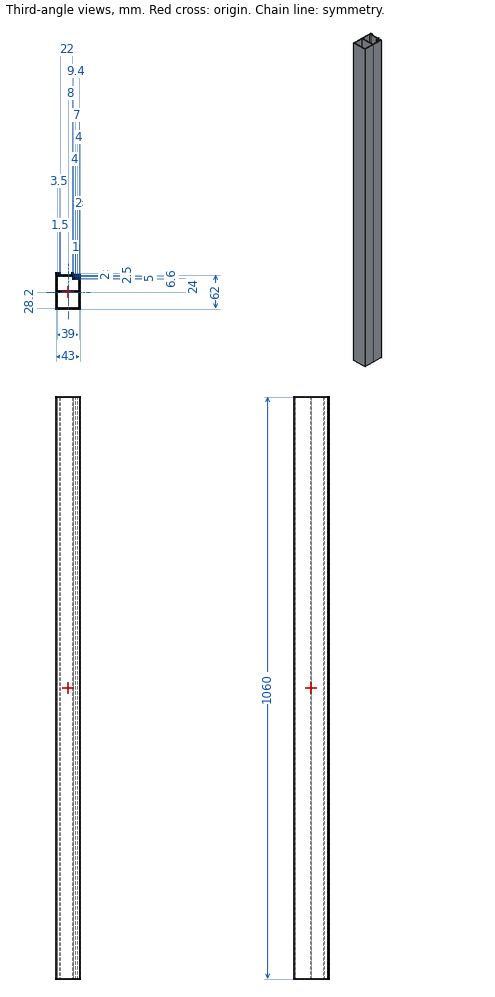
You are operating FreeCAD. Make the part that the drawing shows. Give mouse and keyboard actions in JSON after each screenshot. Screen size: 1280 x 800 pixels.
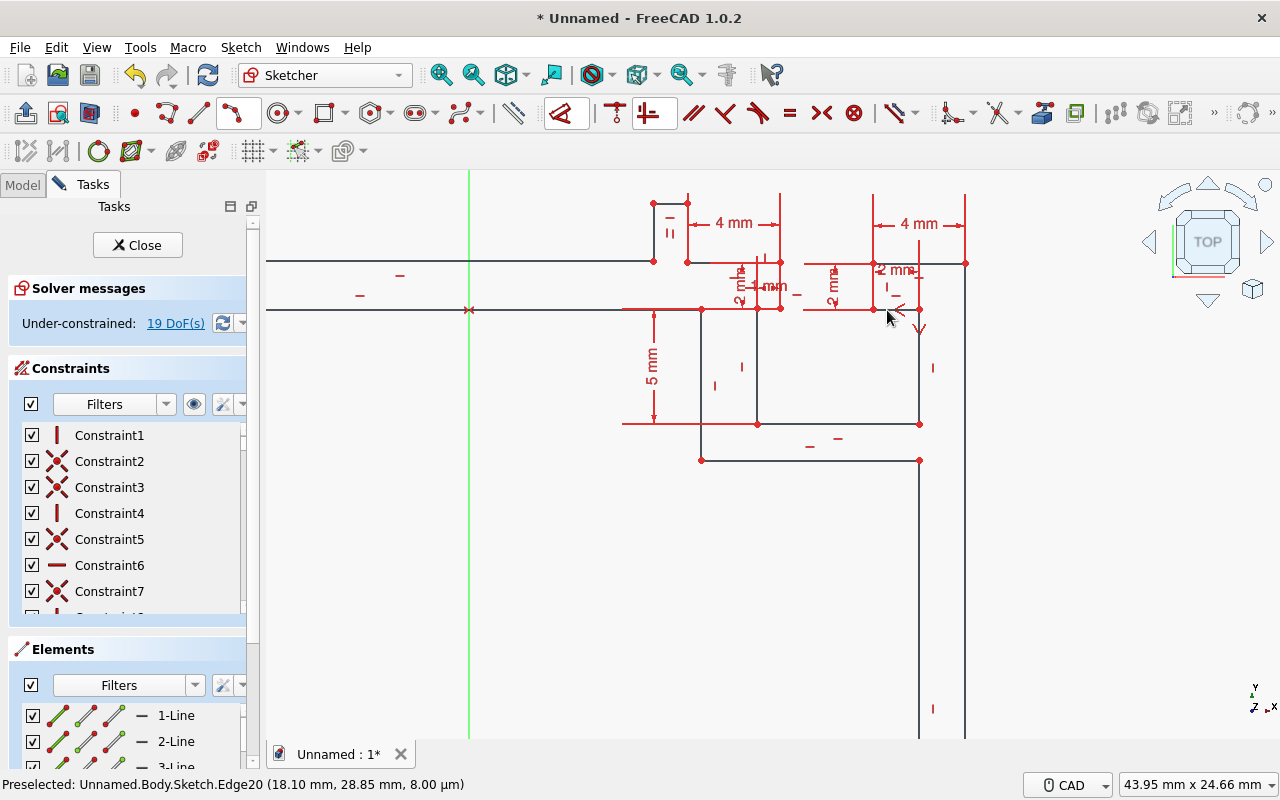
{"action": "left_click", "coordinate": [919, 344]}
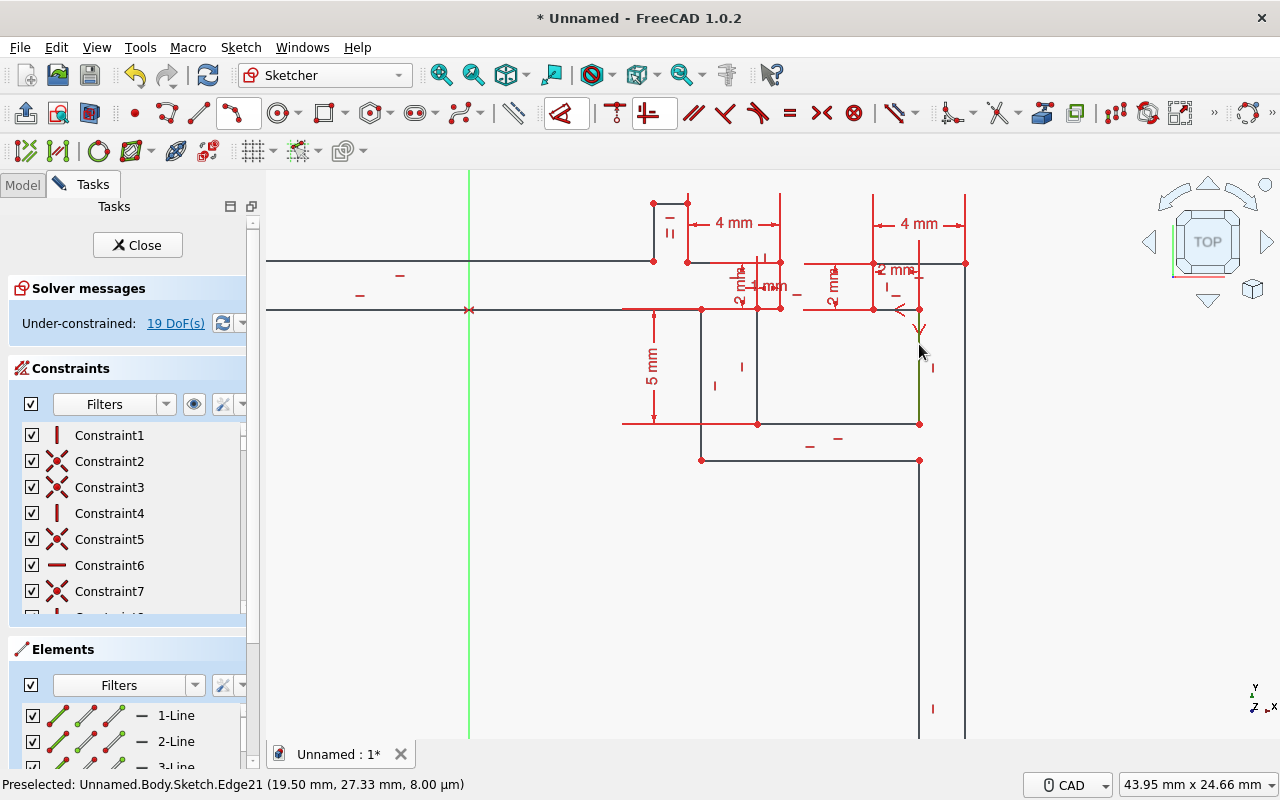
{"action": "key", "text": "i"}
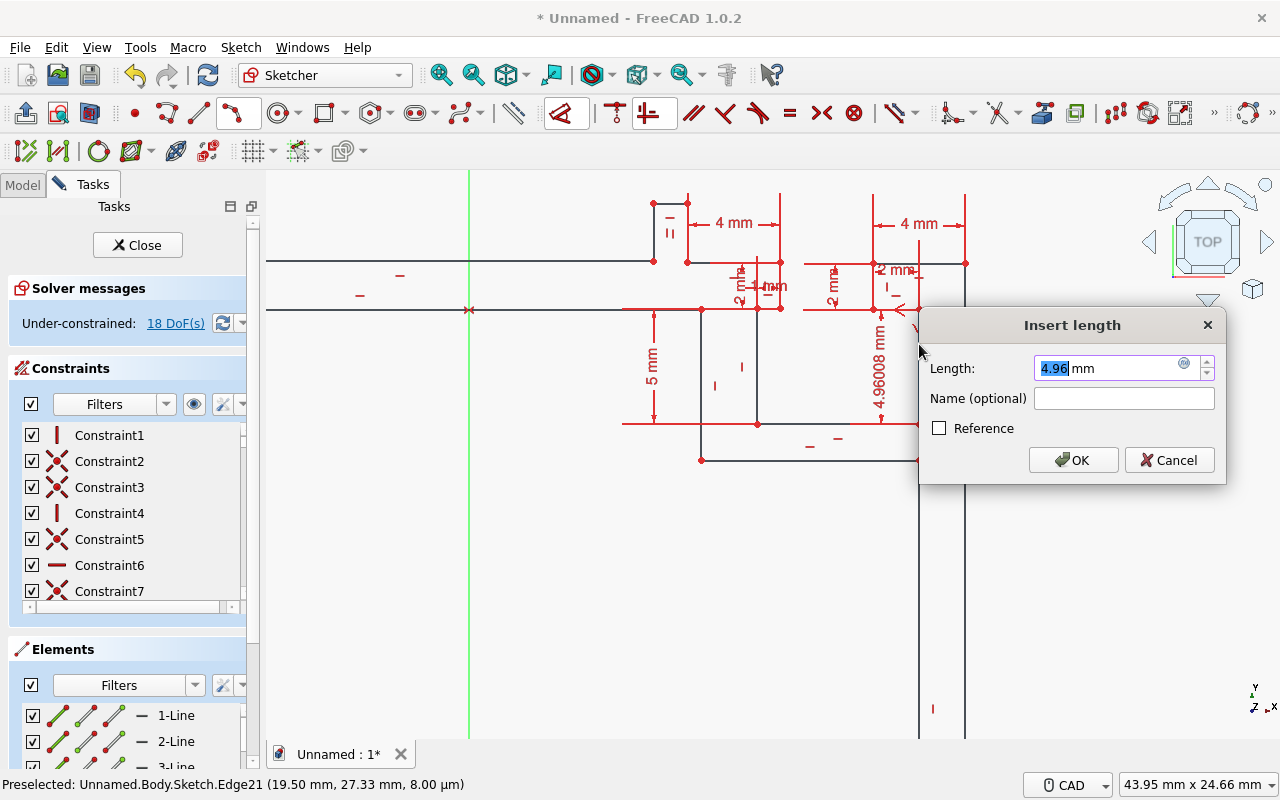
{"action": "type", "text": "5"}
{"action": "key", "text": "Return"}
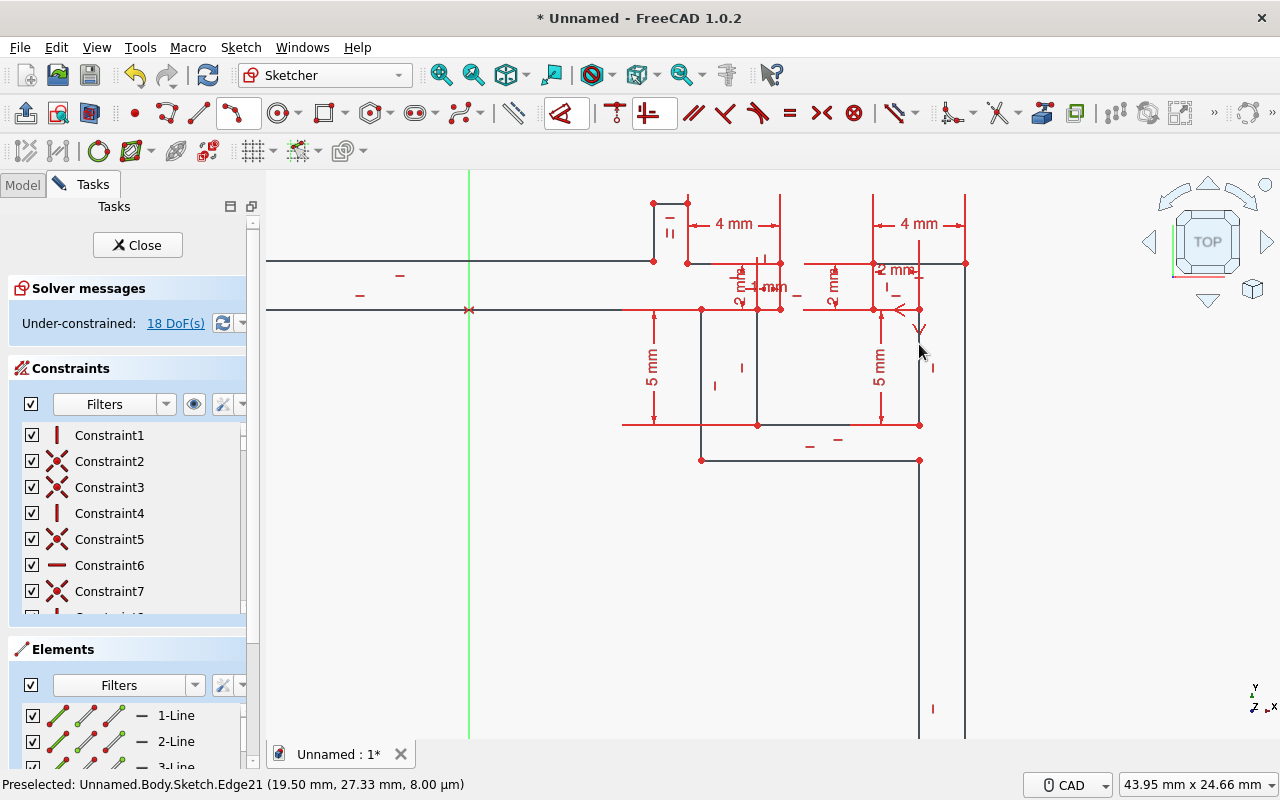
{"action": "left_click", "coordinate": [871, 425]}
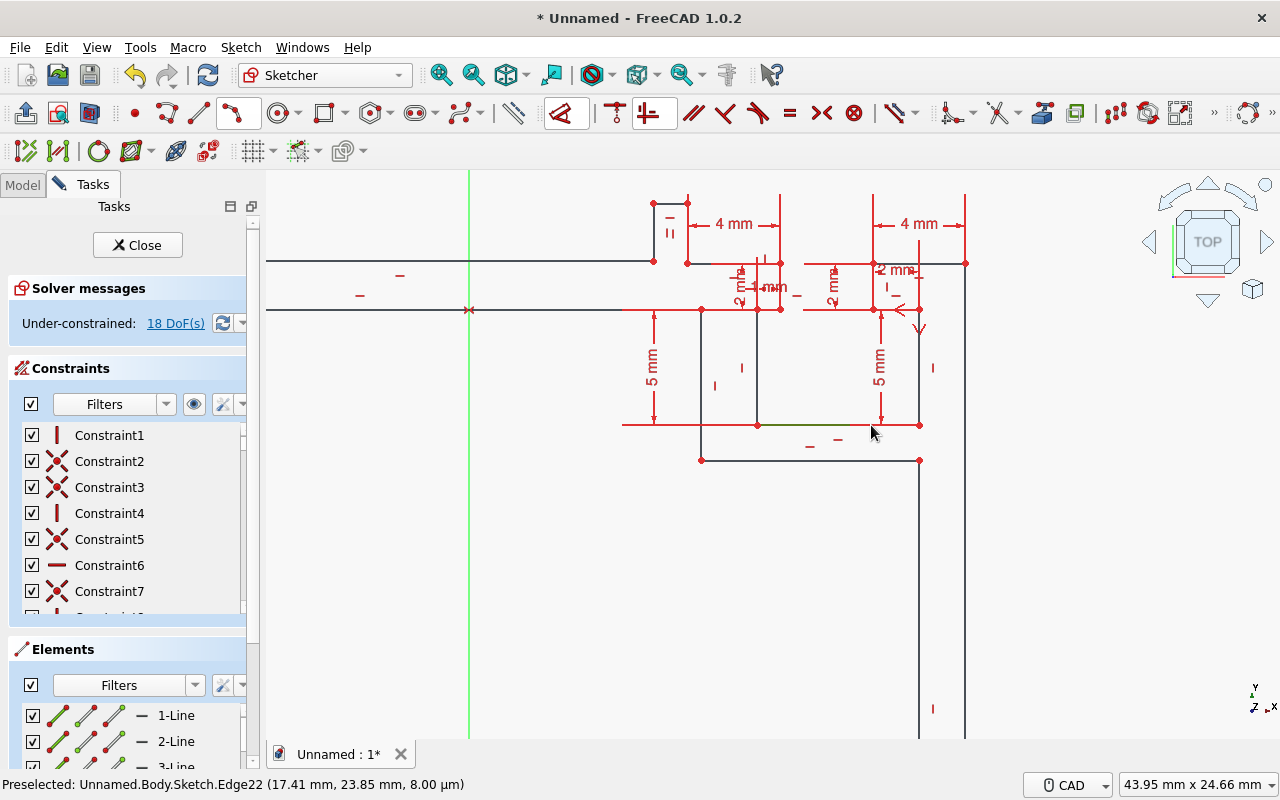
{"action": "left_click", "coordinate": [584, 114]}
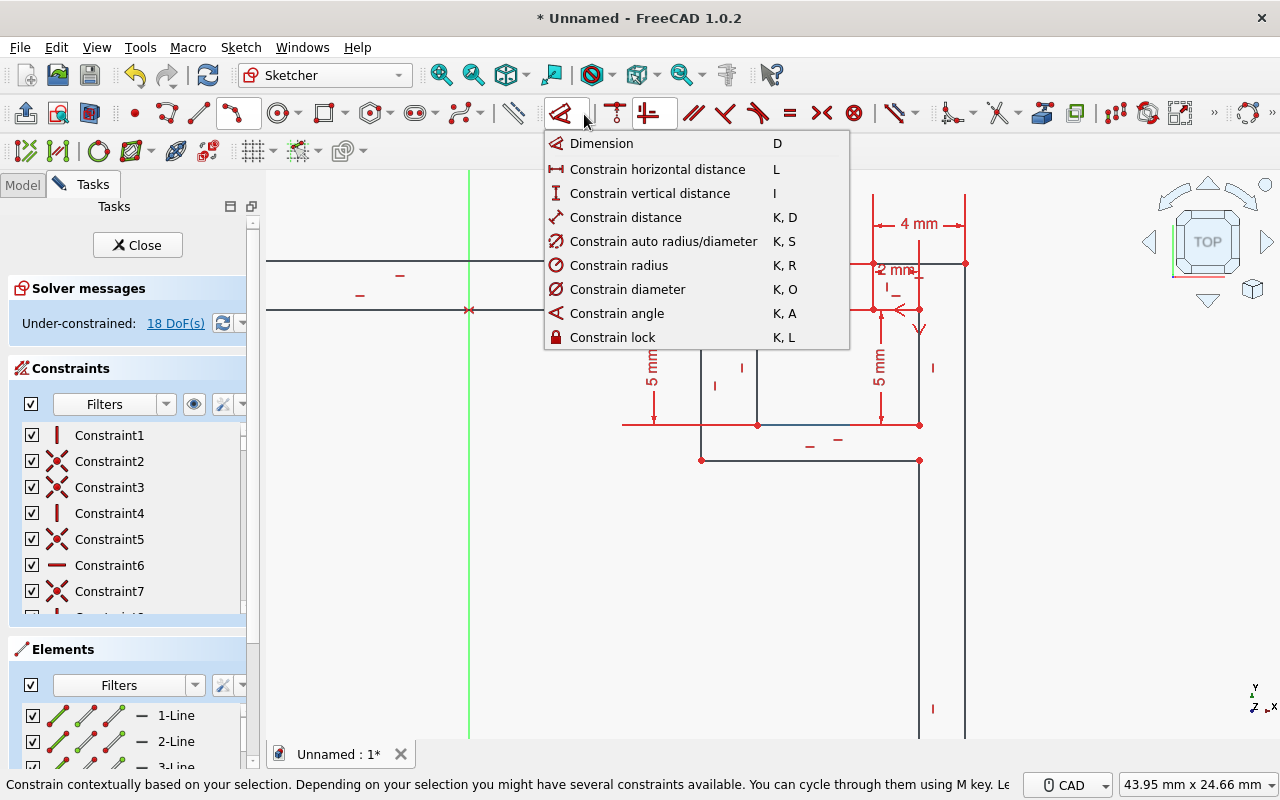
{"action": "left_click", "coordinate": [697, 169]}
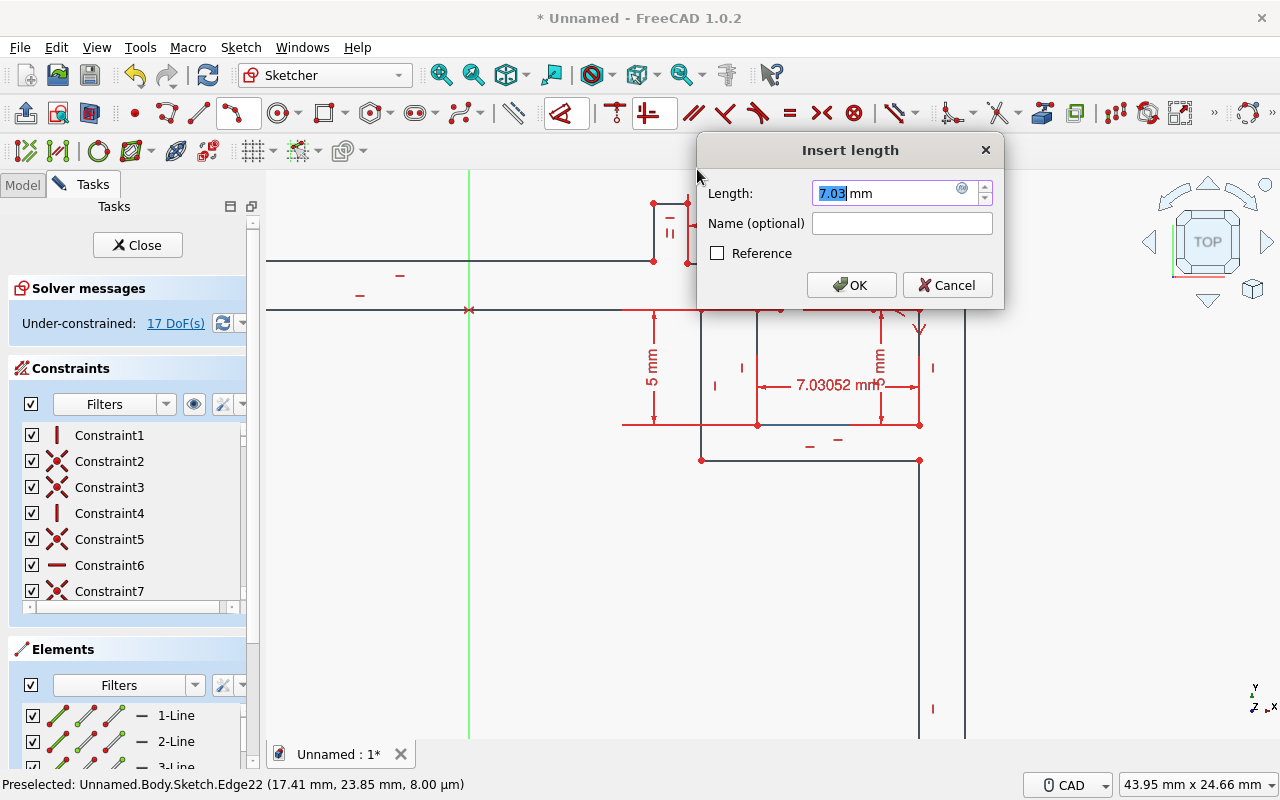
{"action": "type", "text": "7"}
{"action": "key", "text": "Return"}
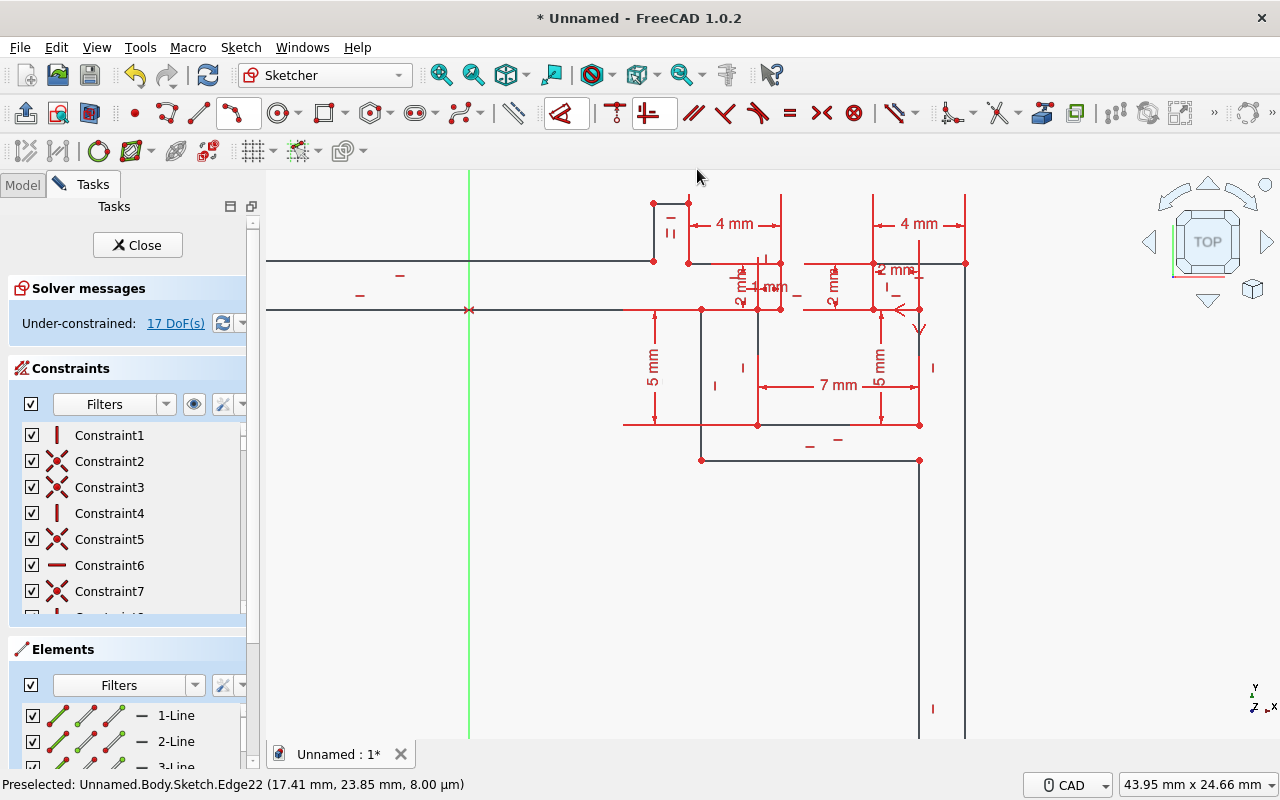
{"action": "left_click", "coordinate": [502, 261]}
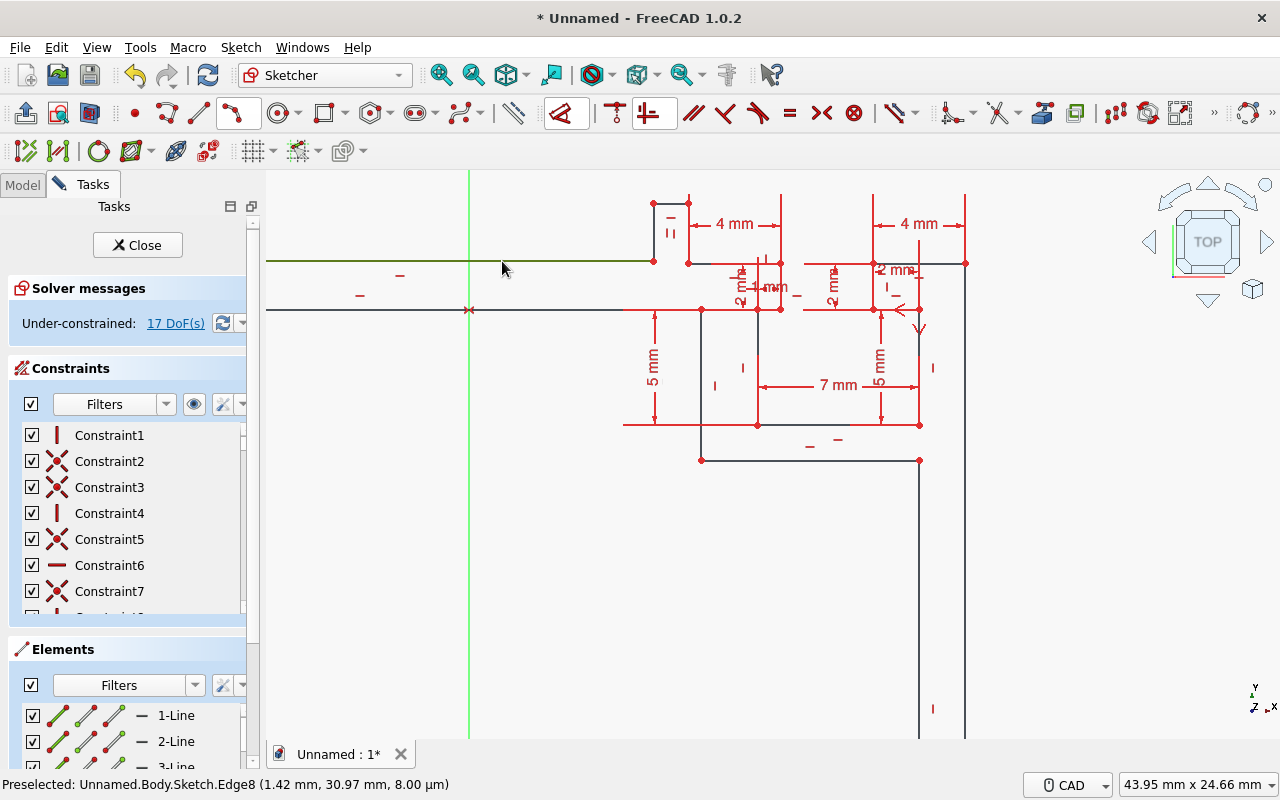
{"action": "key", "text": "l"}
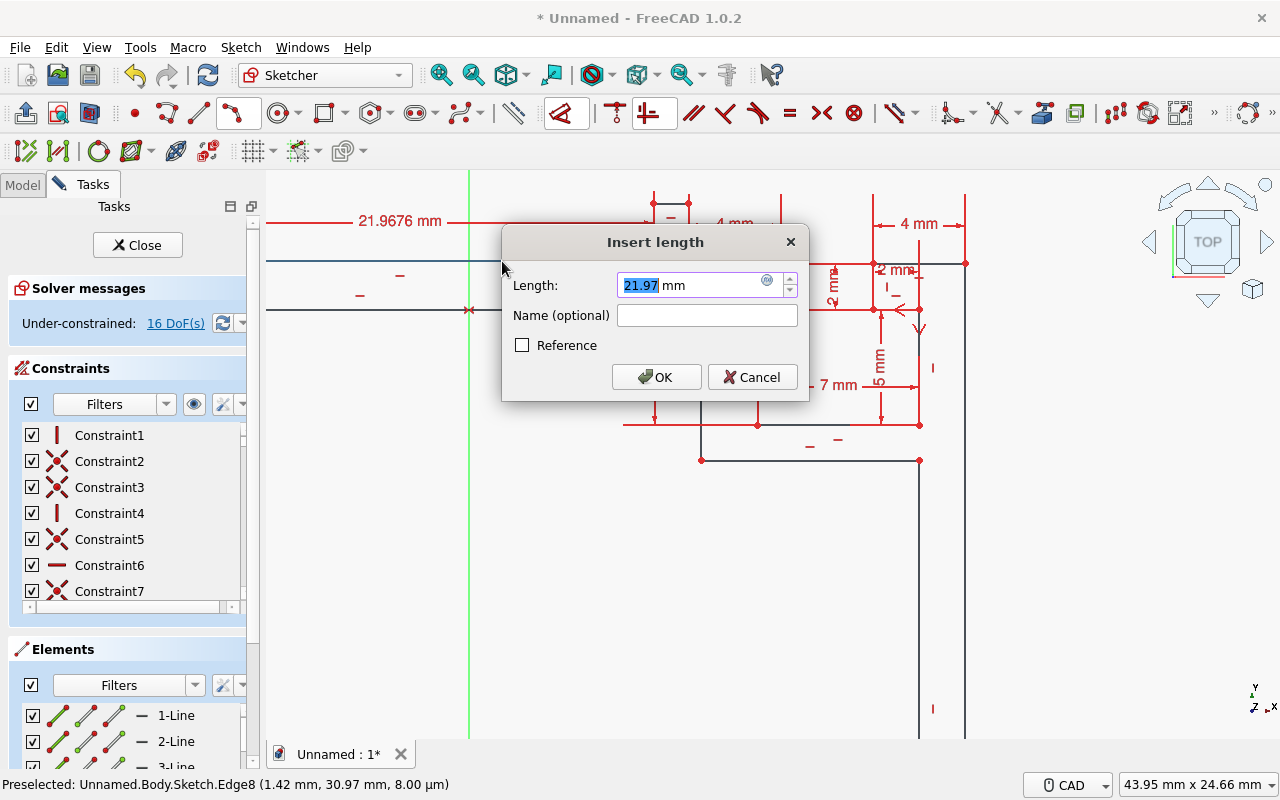
{"action": "type", "text": "22"}
{"action": "key", "text": "Return"}